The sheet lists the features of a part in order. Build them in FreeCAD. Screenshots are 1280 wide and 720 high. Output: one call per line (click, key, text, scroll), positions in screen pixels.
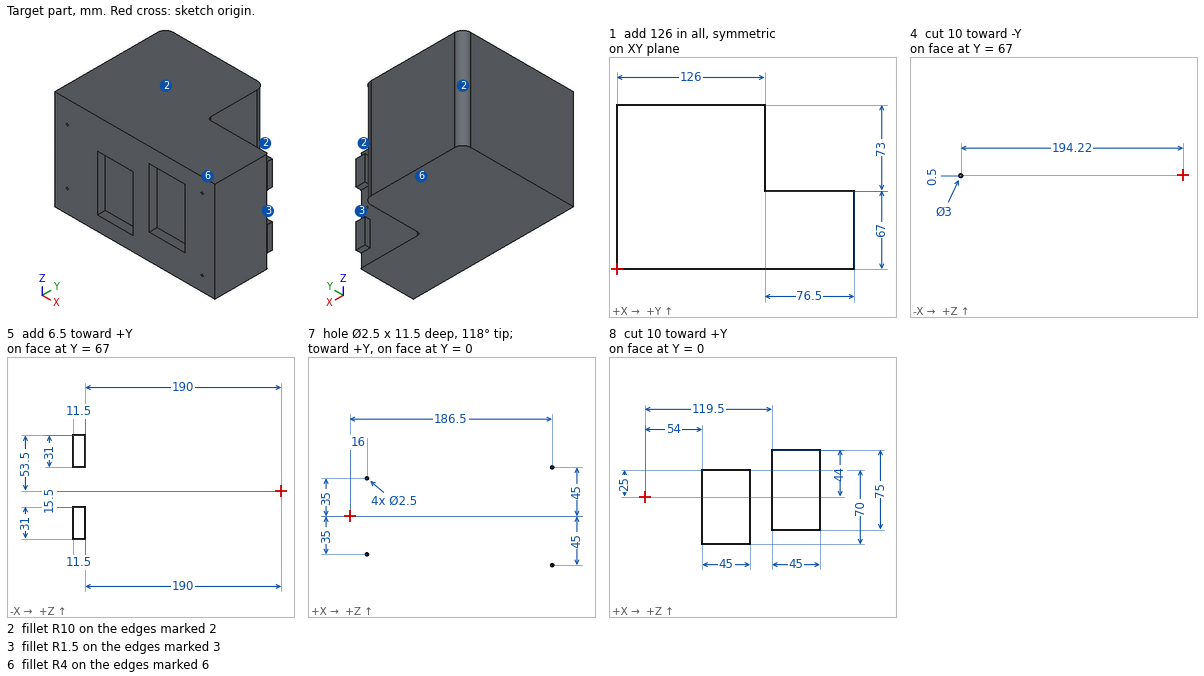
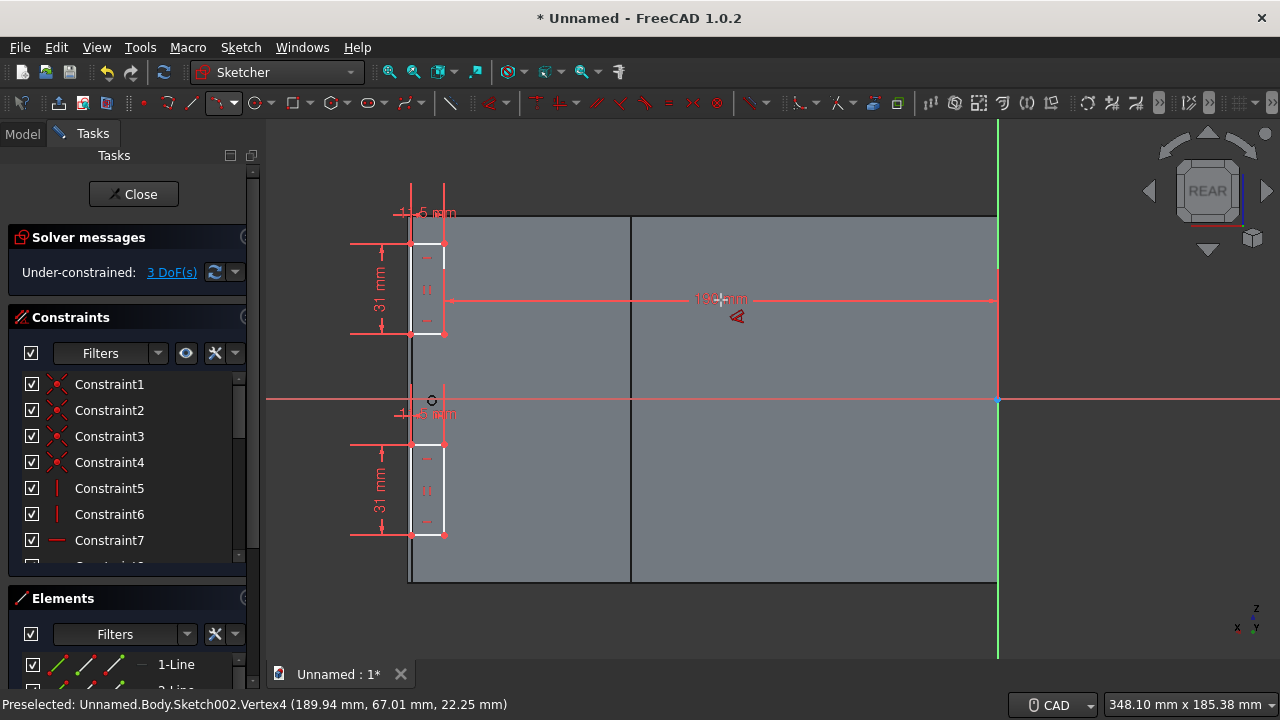
click(444, 535)
click(721, 569)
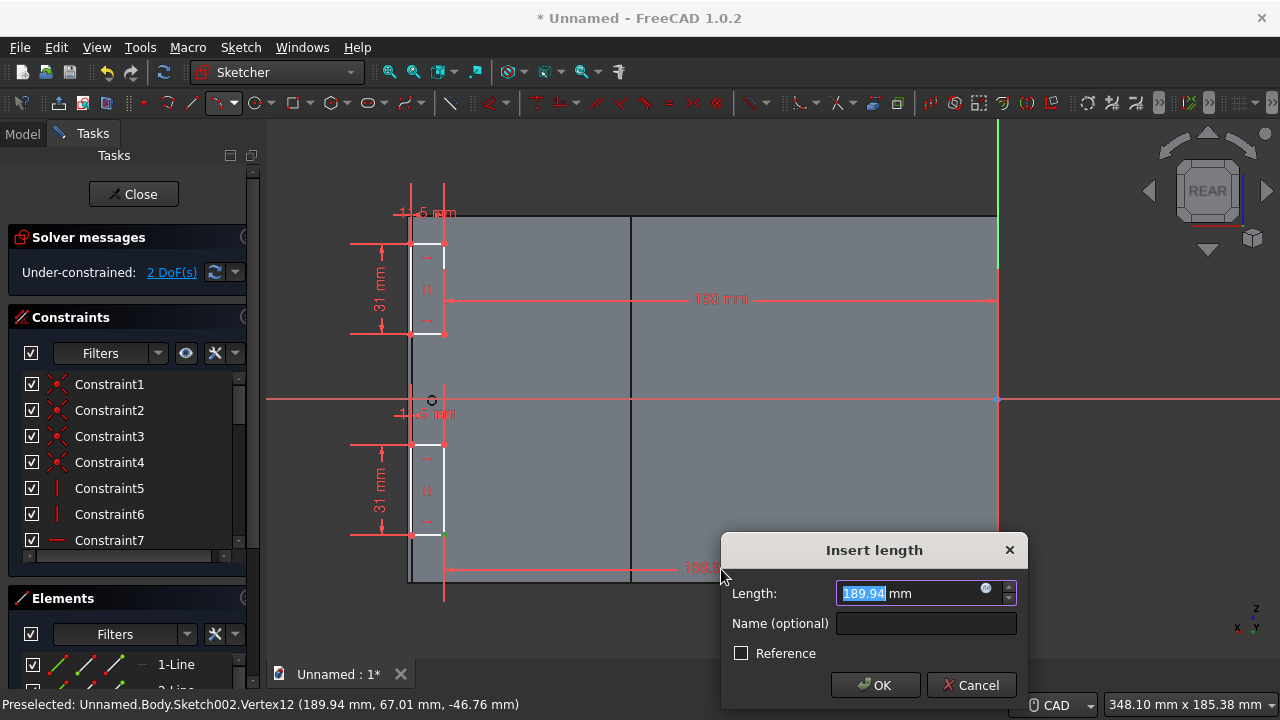
text(190)
key(Return)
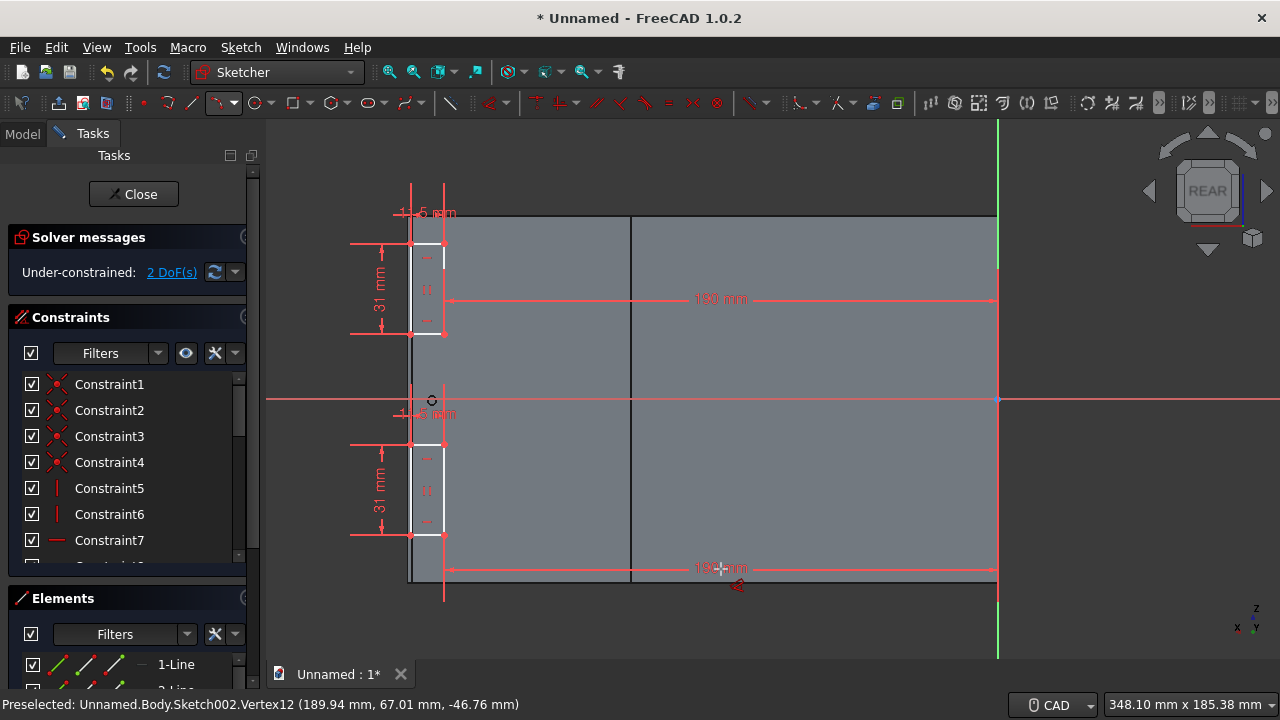
click(411, 244)
click(1032, 322)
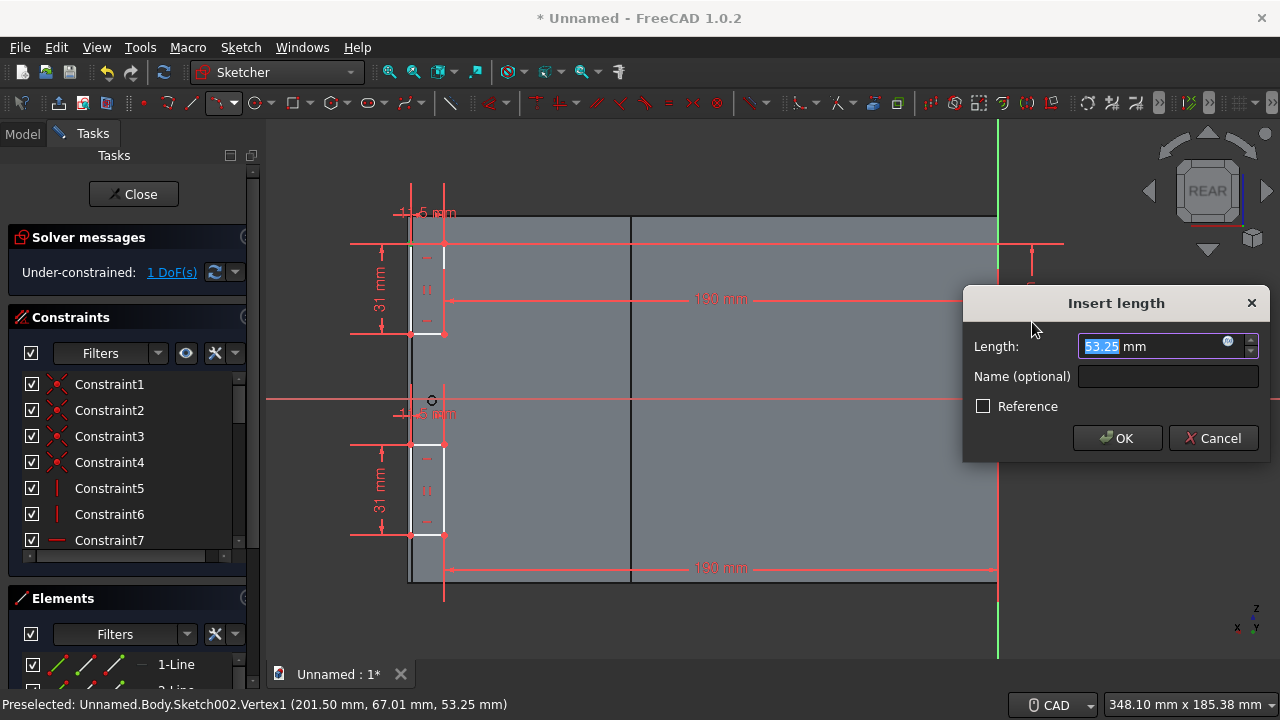
text(53.5)
key(Return)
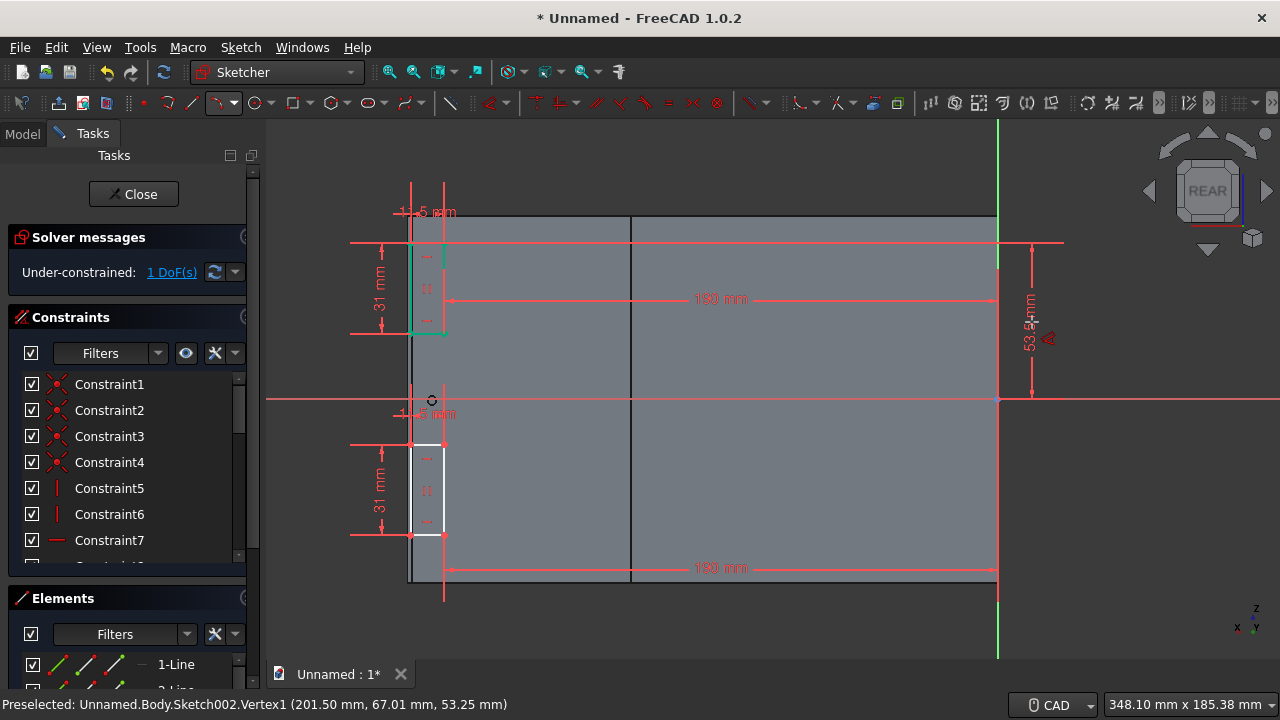
click(411, 445)
click(1032, 422)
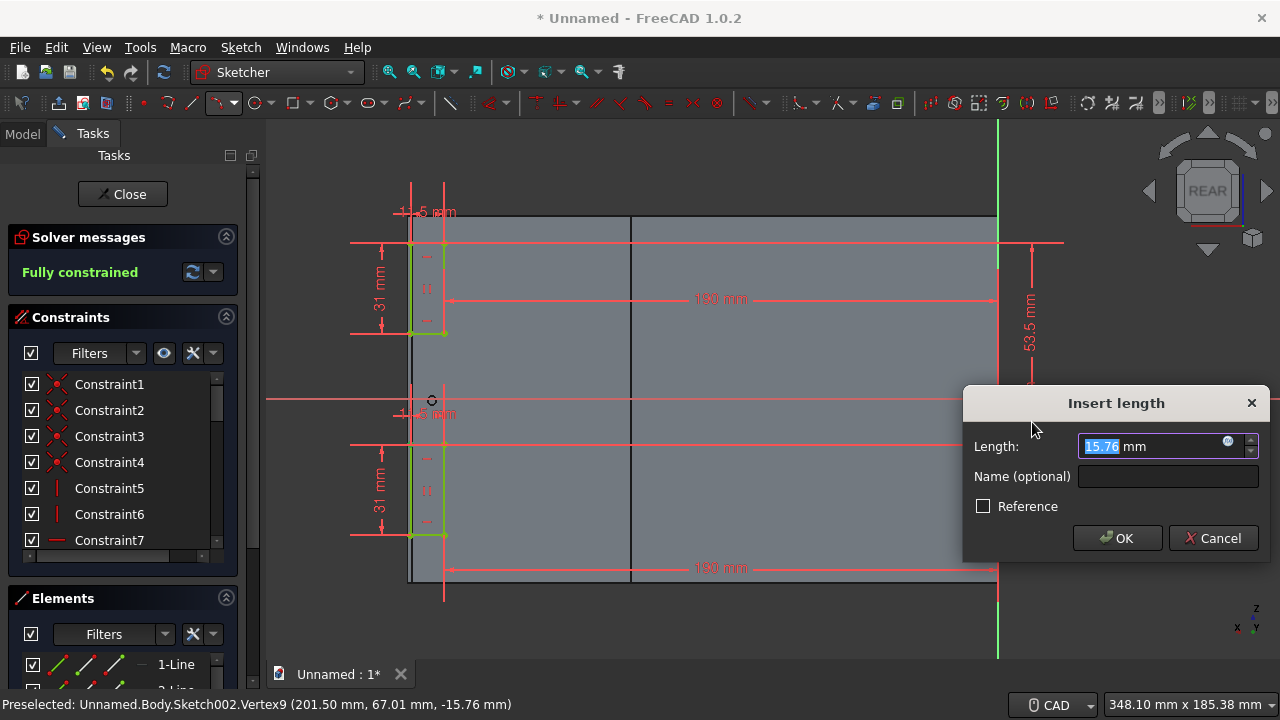
text(15.5)
key(Return)
key(Escape)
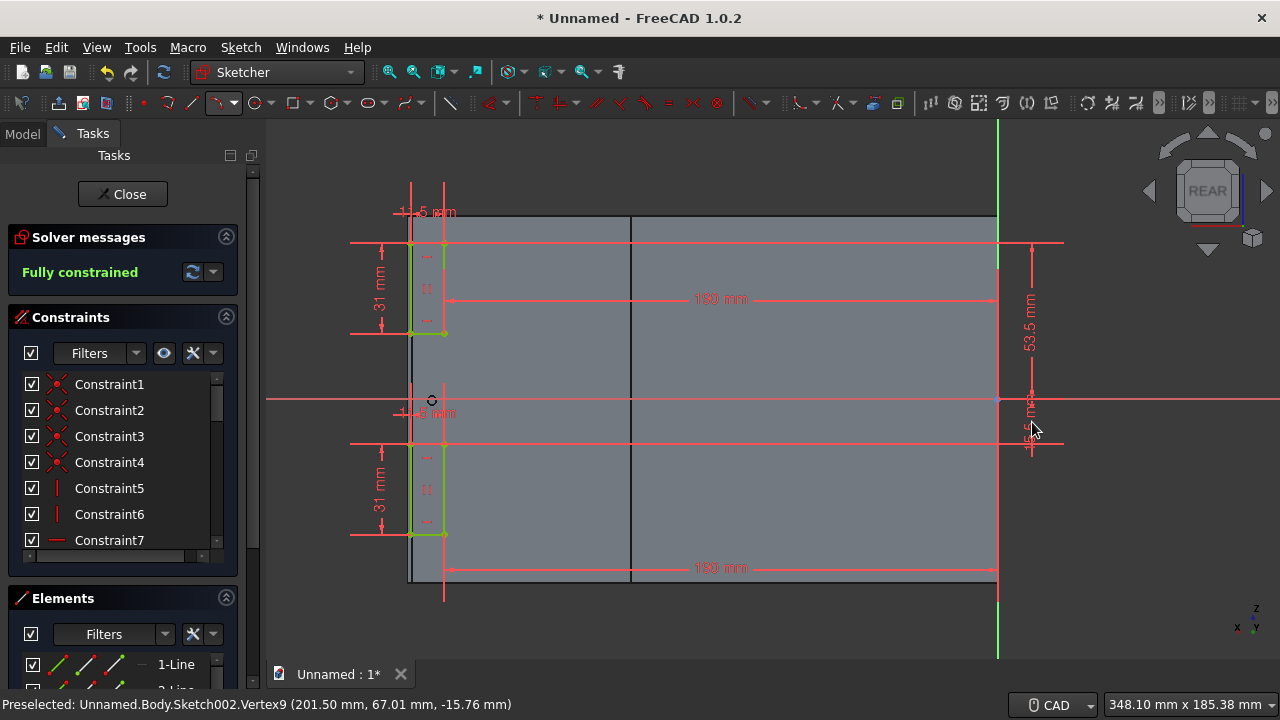
click(123, 194)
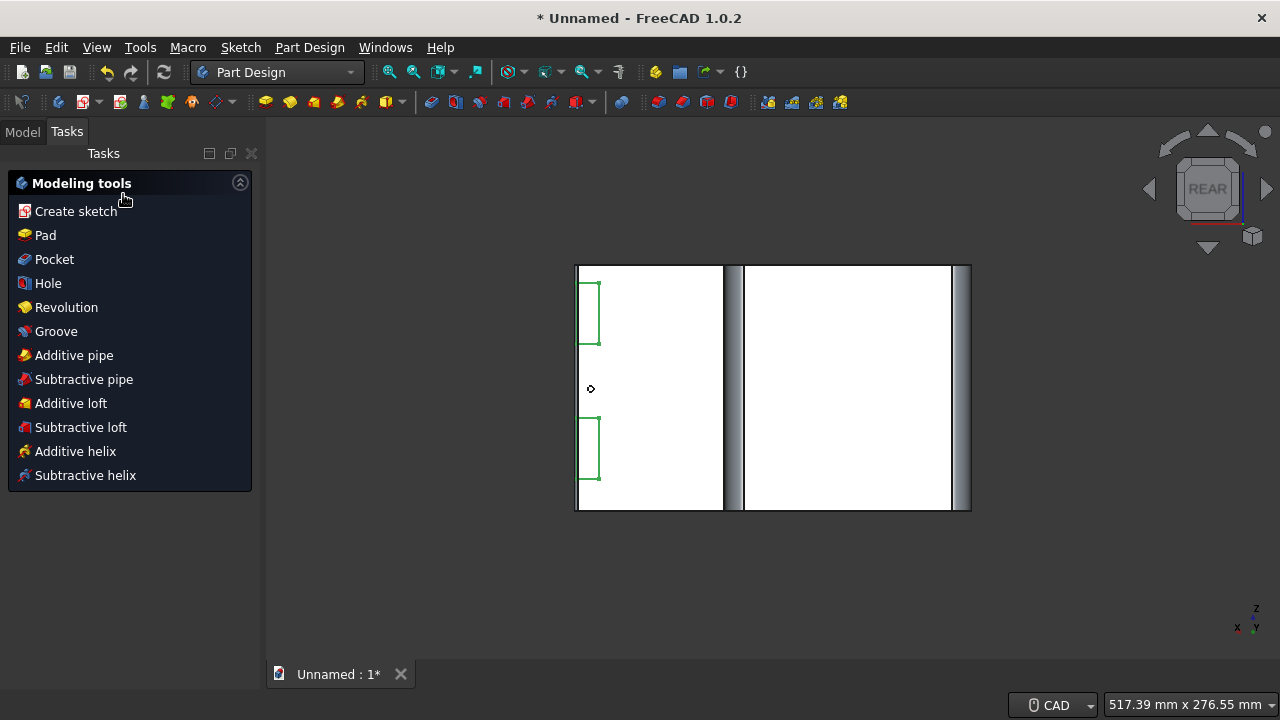
click(266, 102)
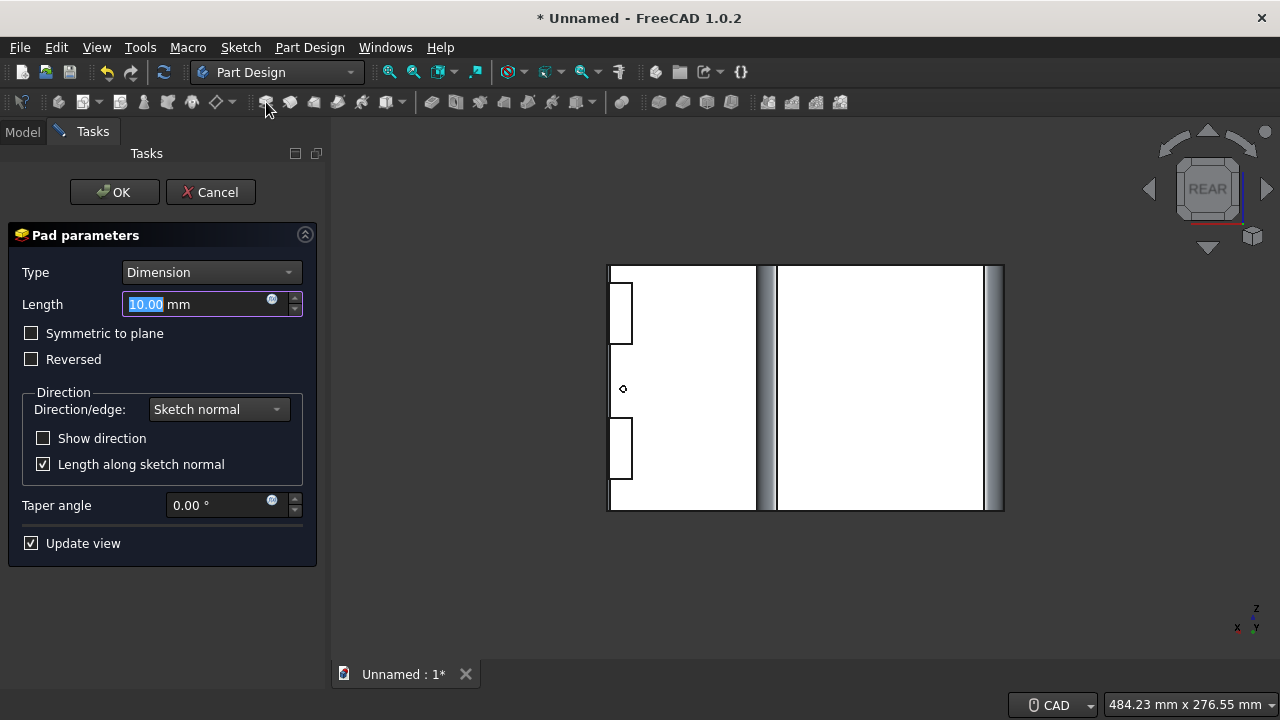
text(6.5)
key(Tab)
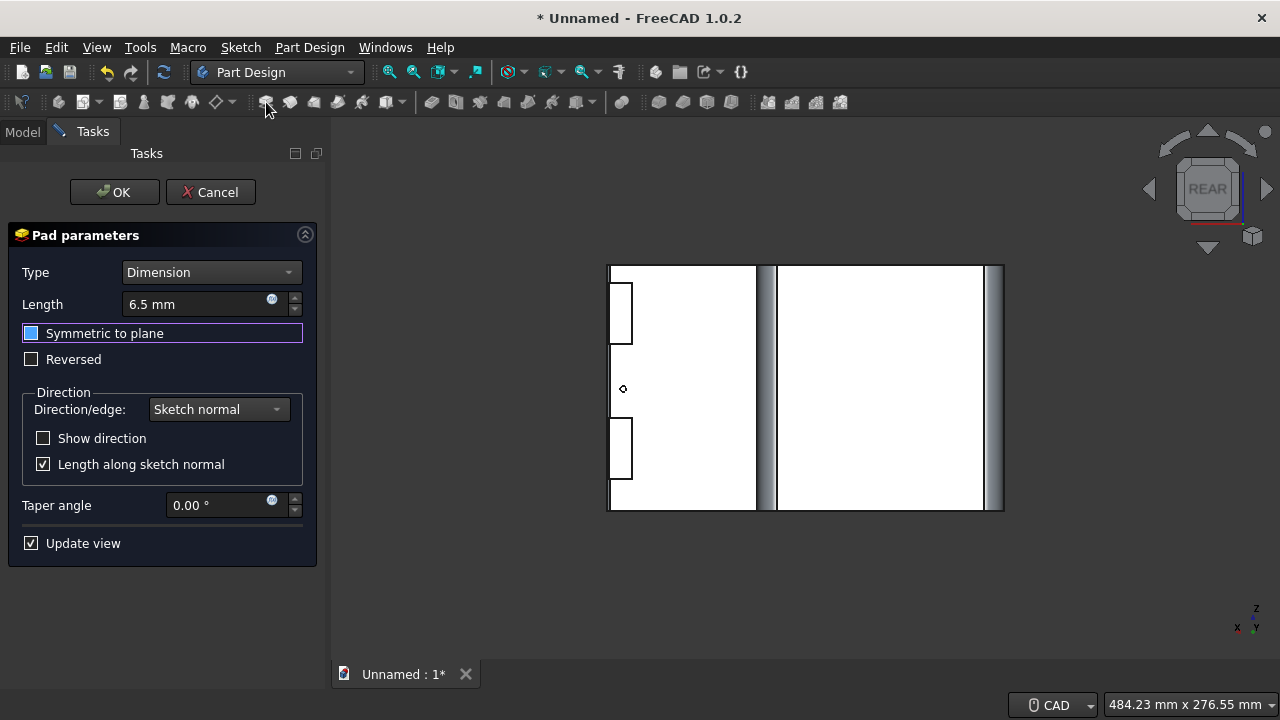
click(115, 192)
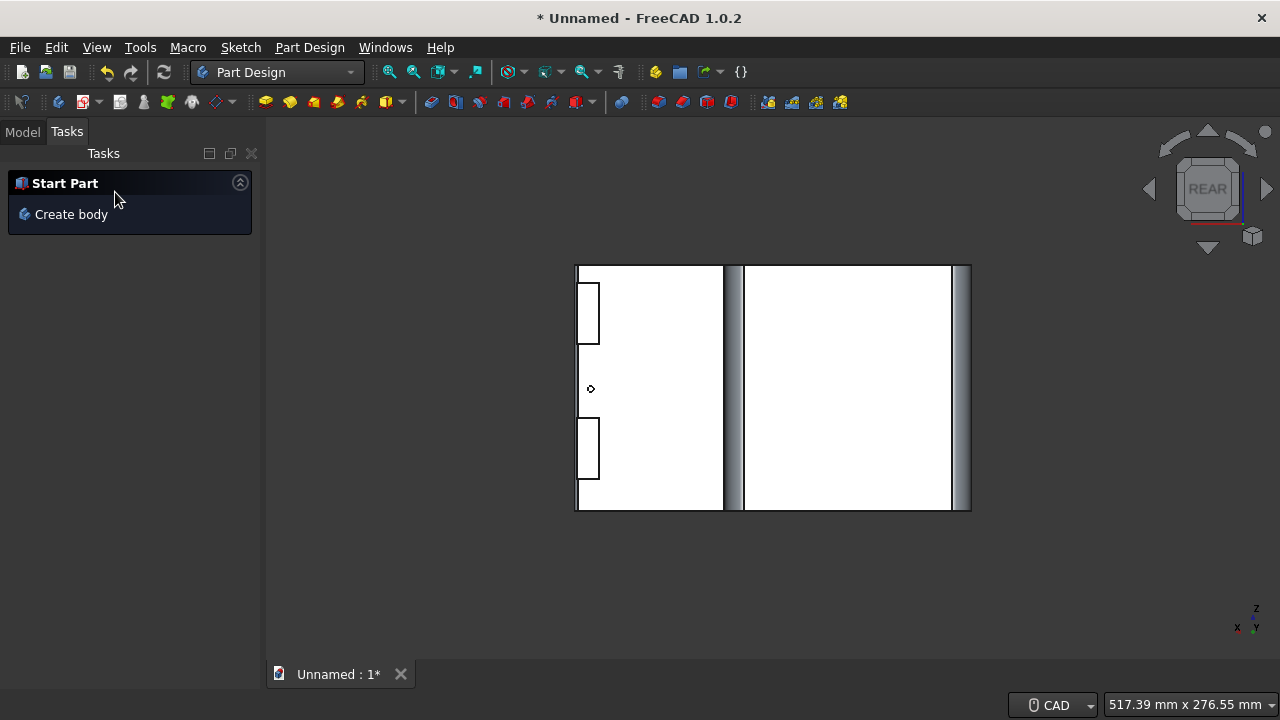
key(0)